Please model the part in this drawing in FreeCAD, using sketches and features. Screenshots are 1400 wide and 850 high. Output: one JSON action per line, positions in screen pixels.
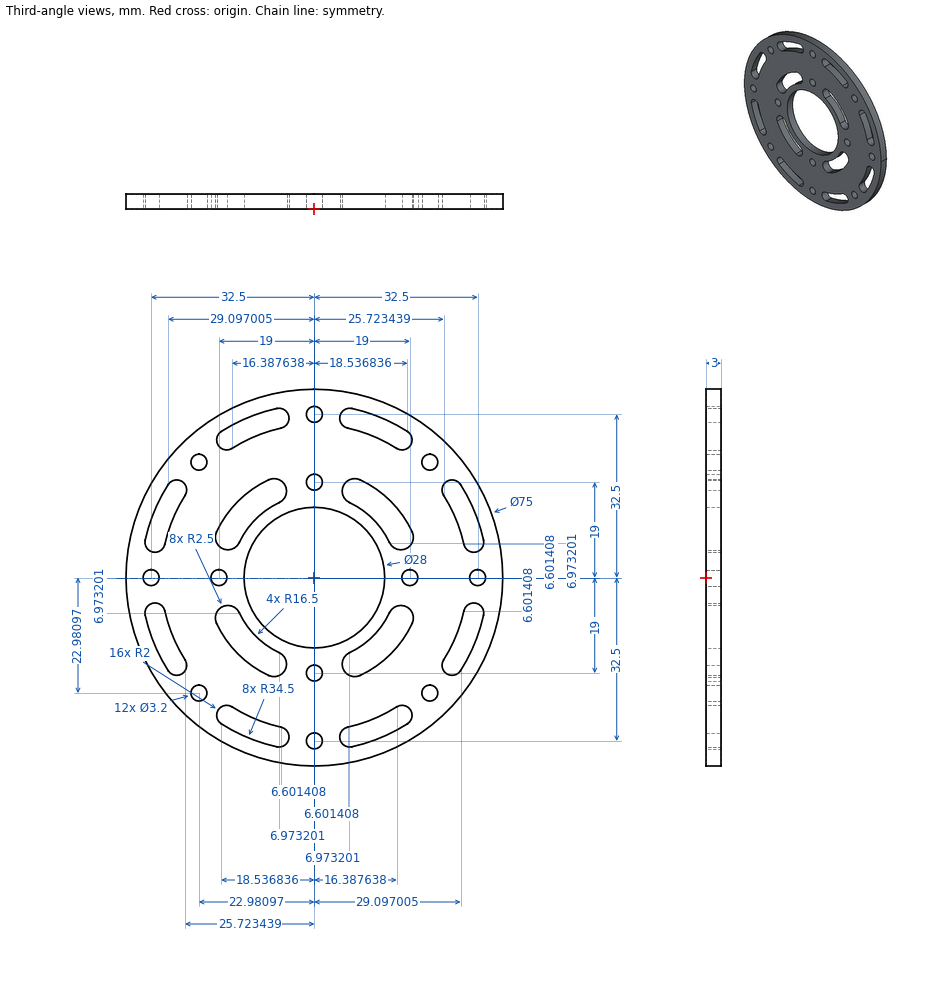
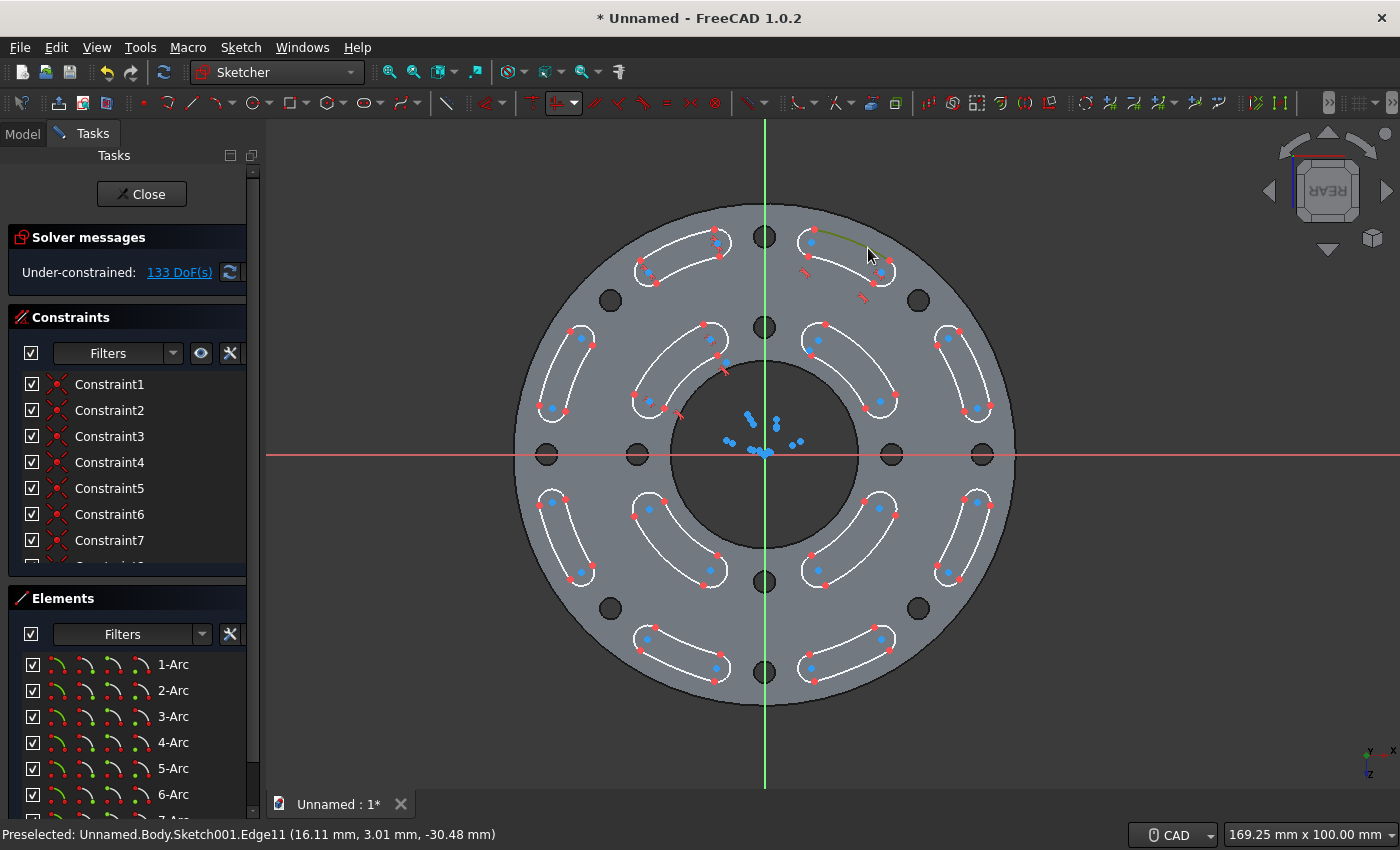
{"action": "left_click", "coordinate": [802, 233]}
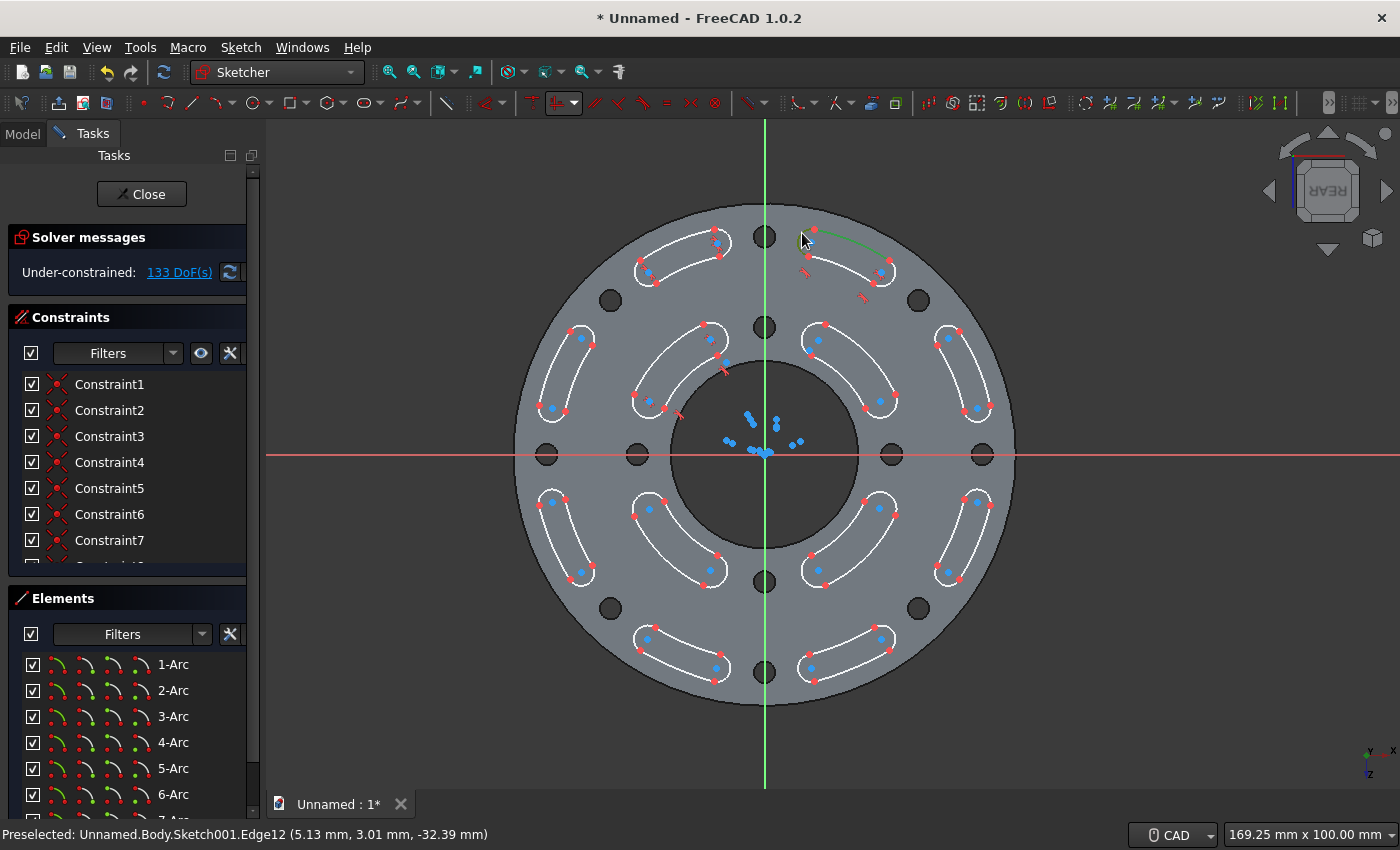
{"action": "left_click", "coordinate": [644, 104]}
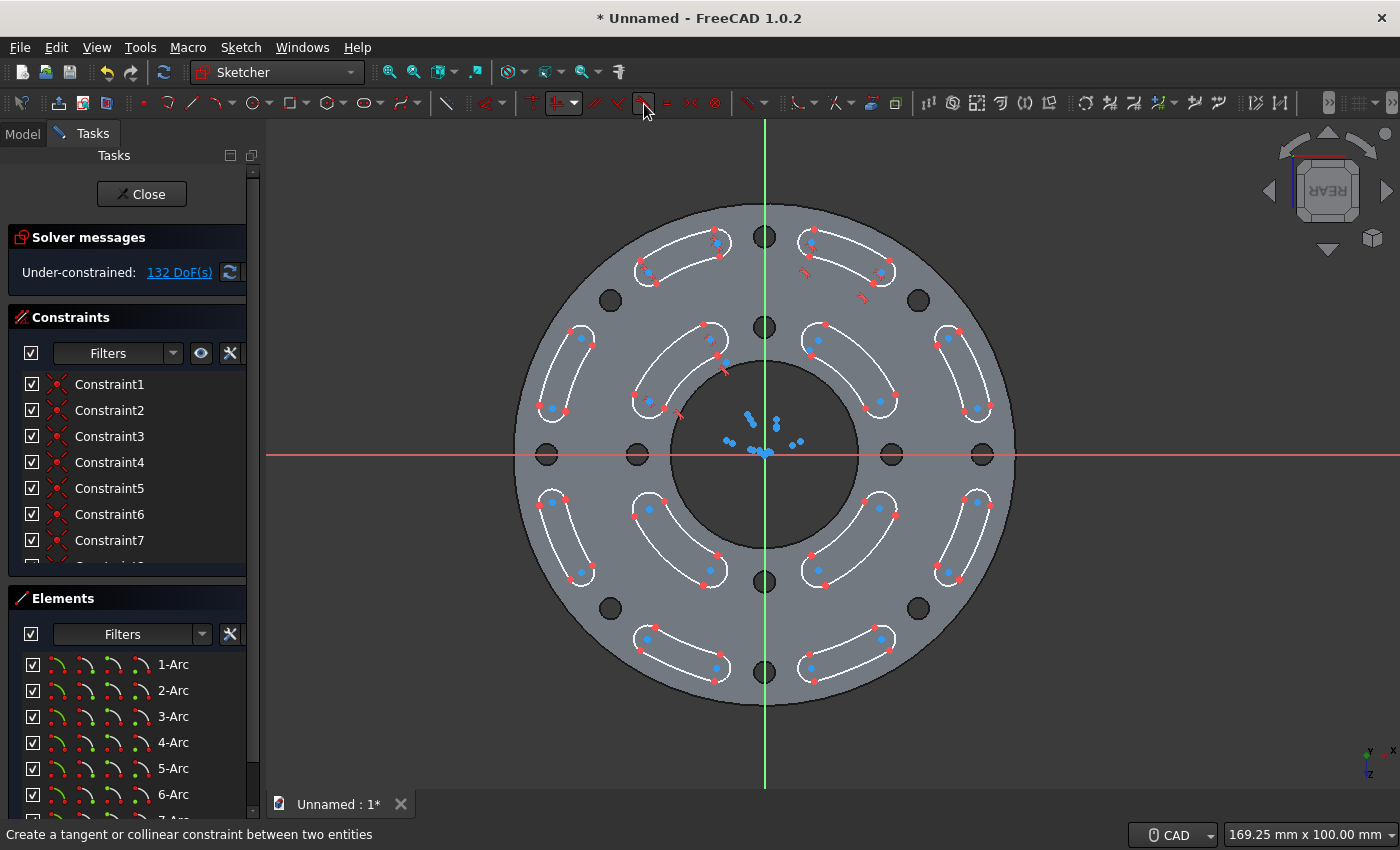
{"action": "left_click", "coordinate": [972, 421]}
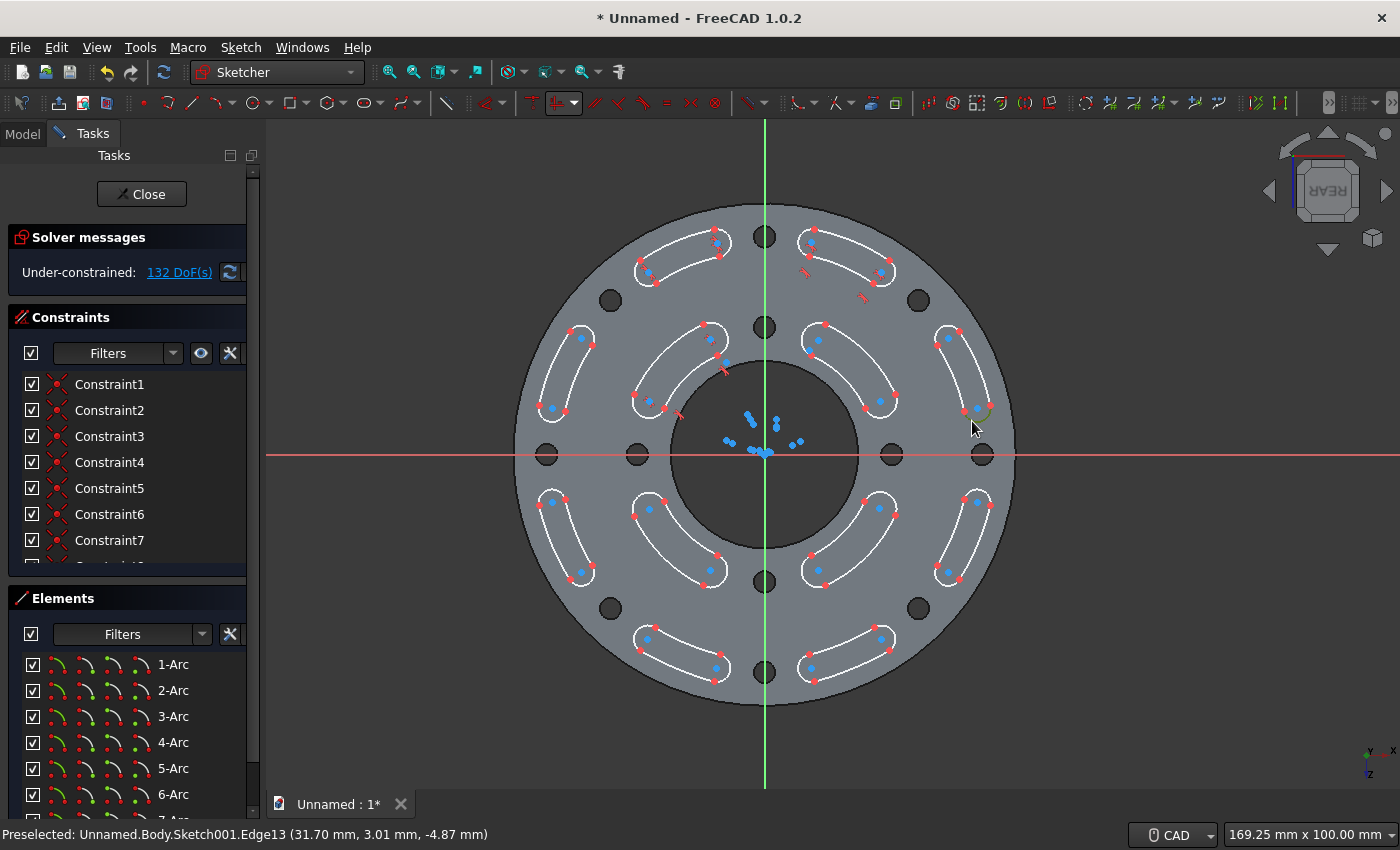
{"action": "left_click", "coordinate": [984, 382]}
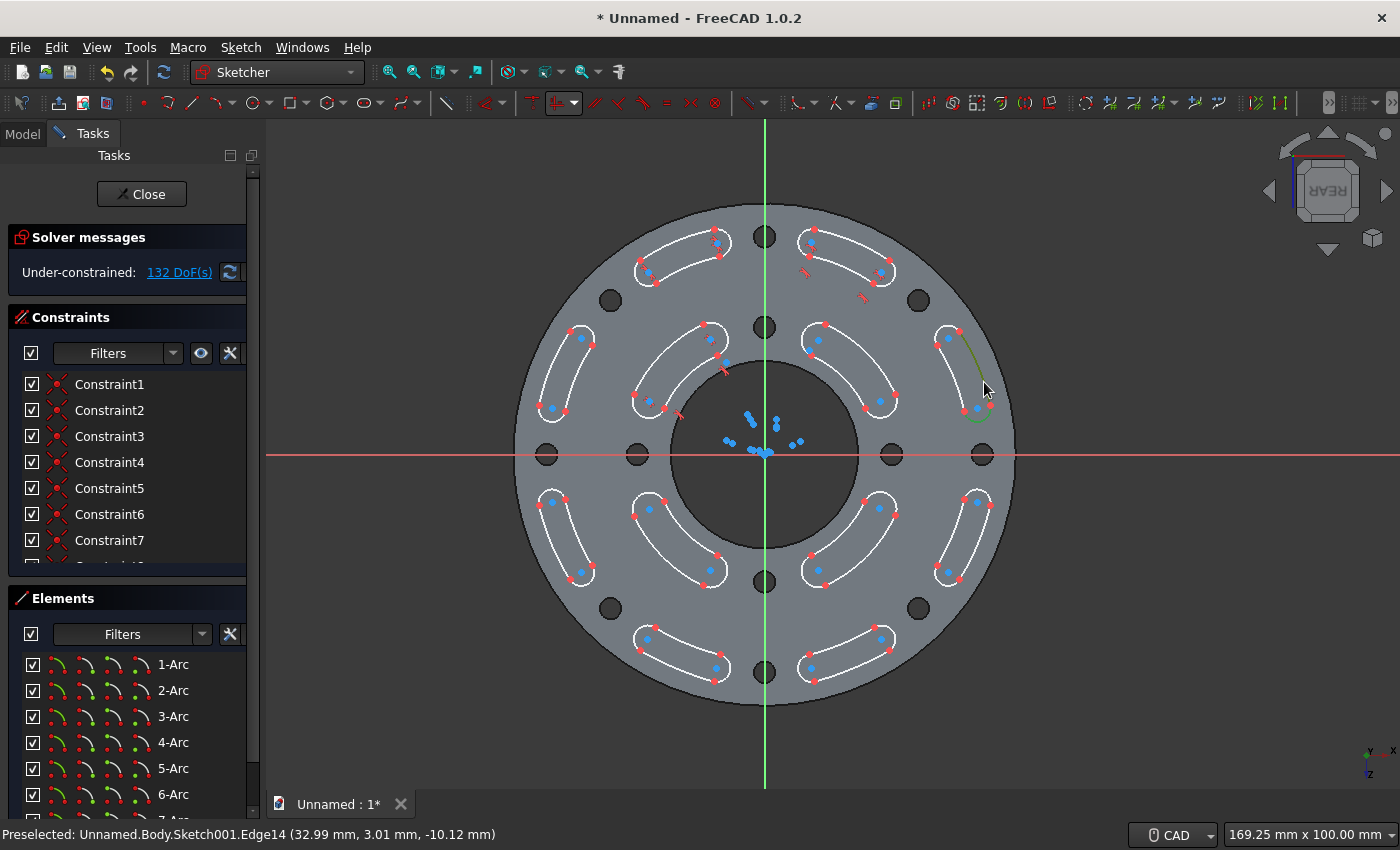
{"action": "left_click", "coordinate": [644, 104]}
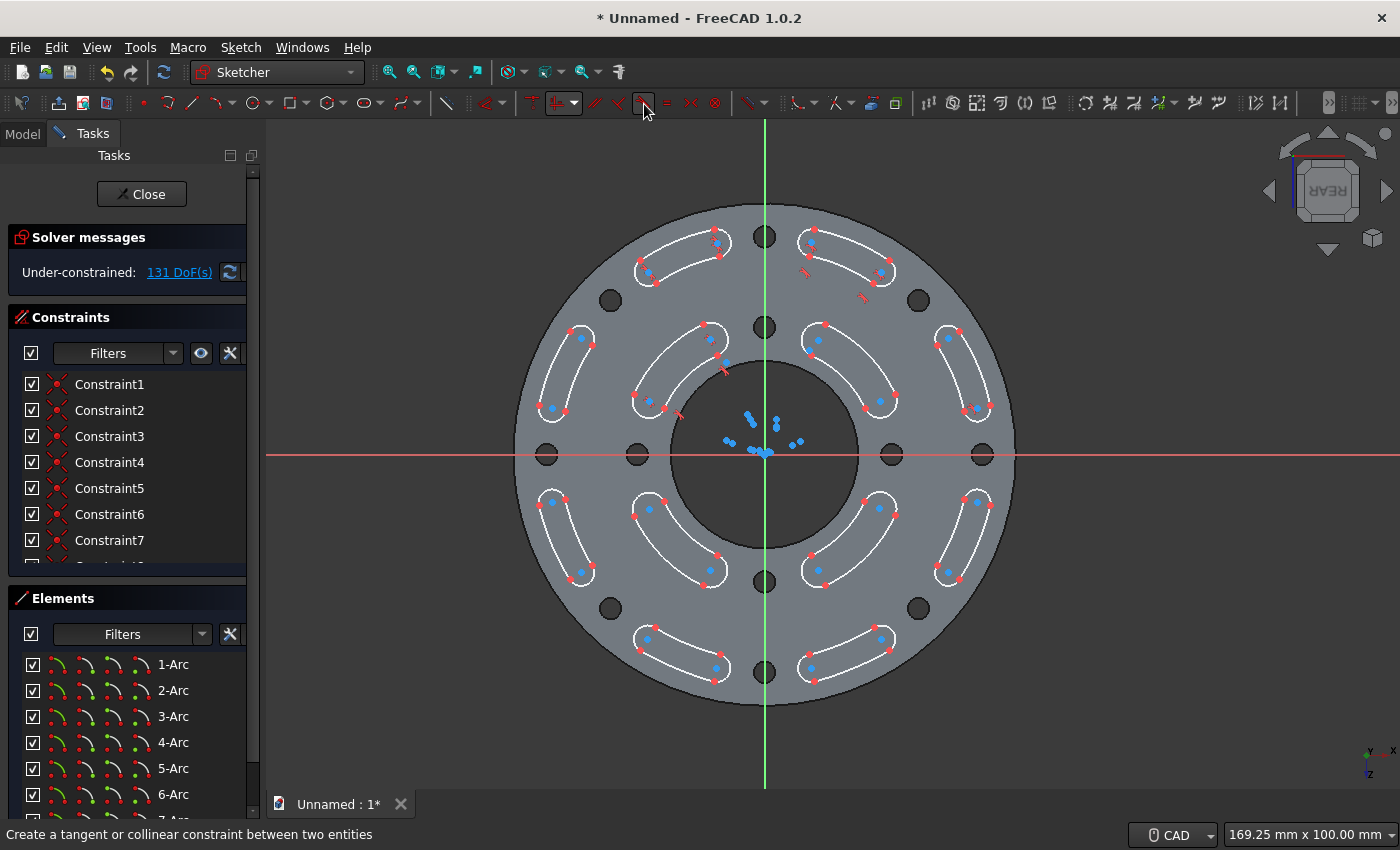
{"action": "left_click", "coordinate": [972, 421]}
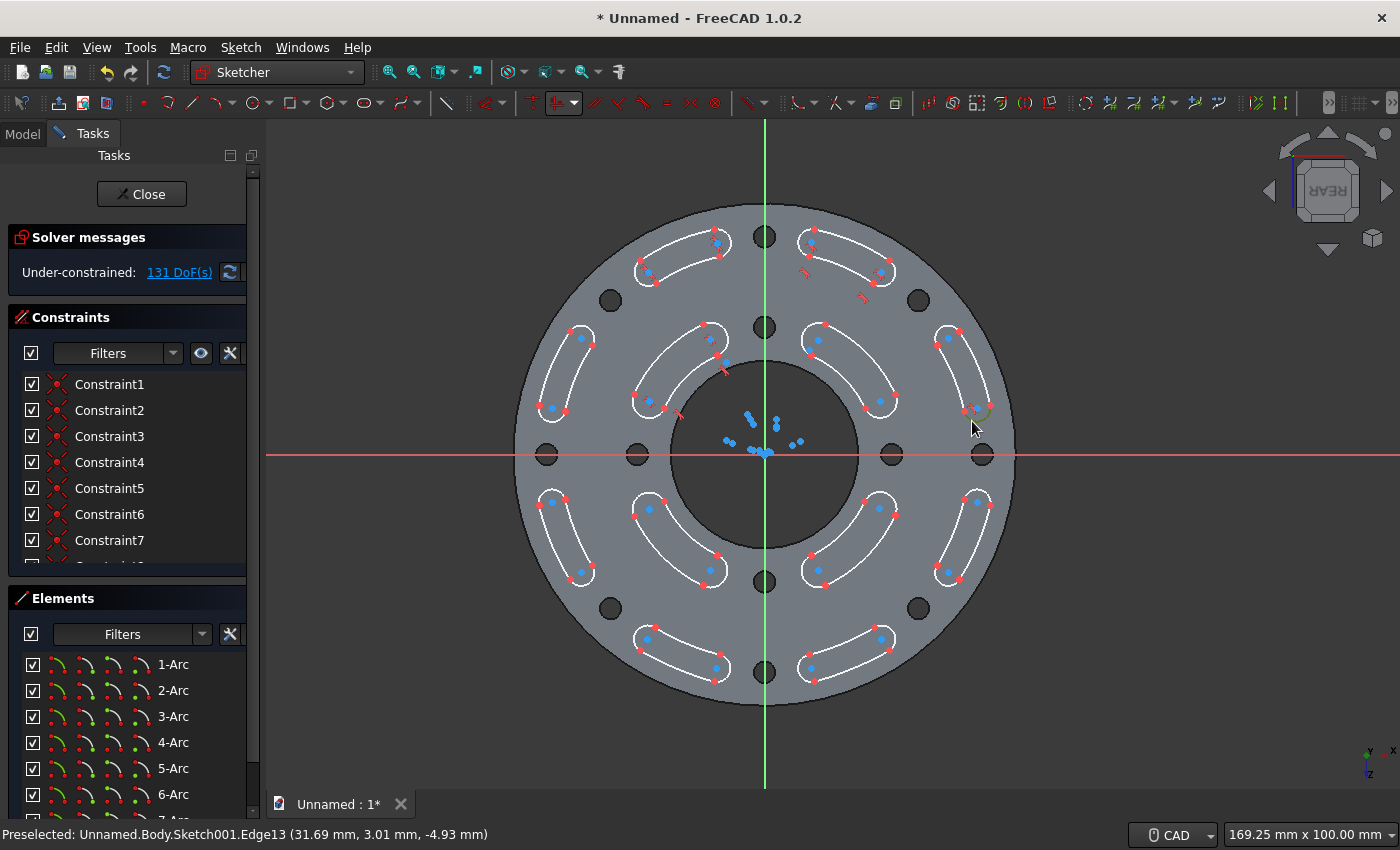
{"action": "left_click", "coordinate": [959, 391]}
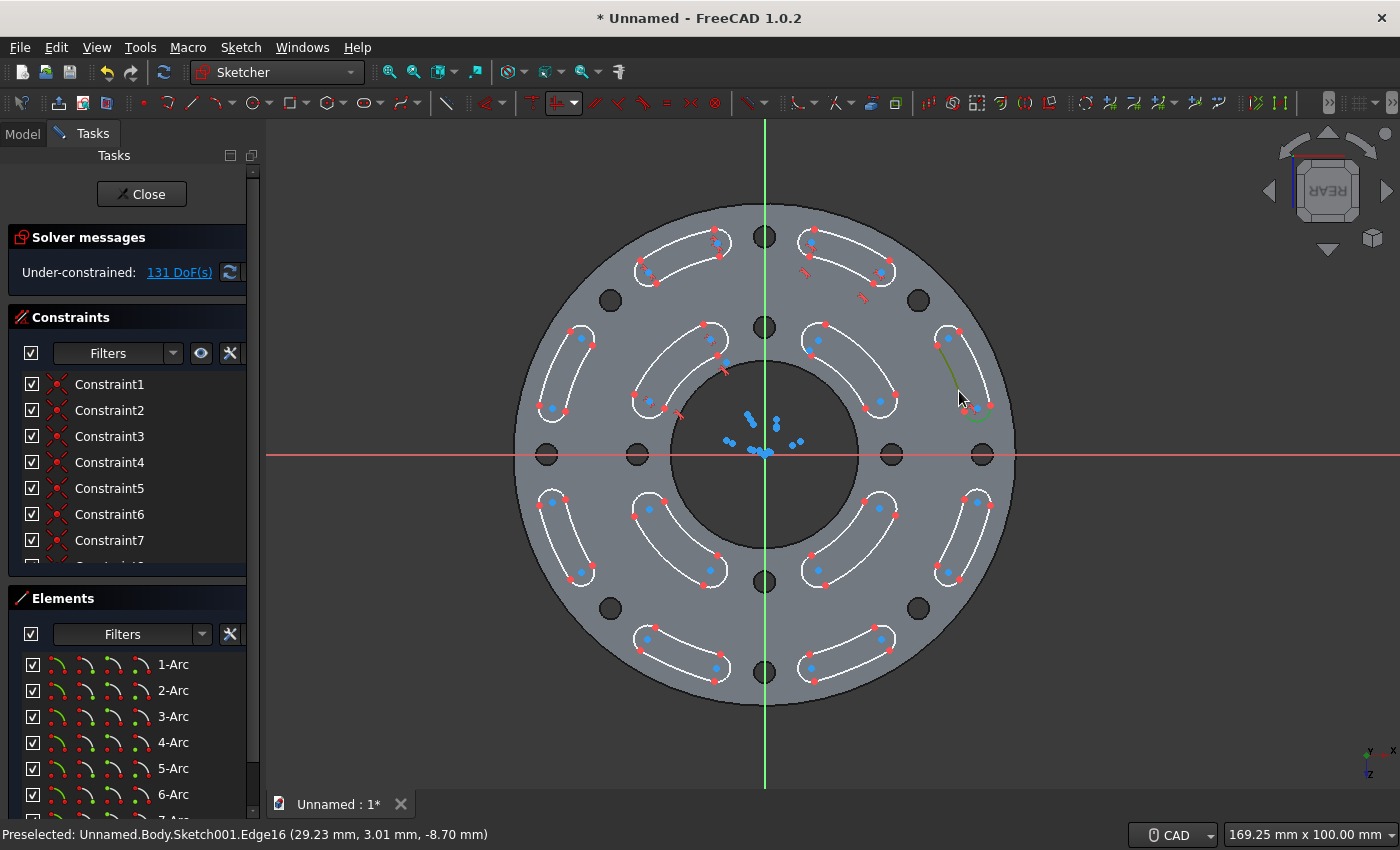
{"action": "left_click", "coordinate": [644, 104]}